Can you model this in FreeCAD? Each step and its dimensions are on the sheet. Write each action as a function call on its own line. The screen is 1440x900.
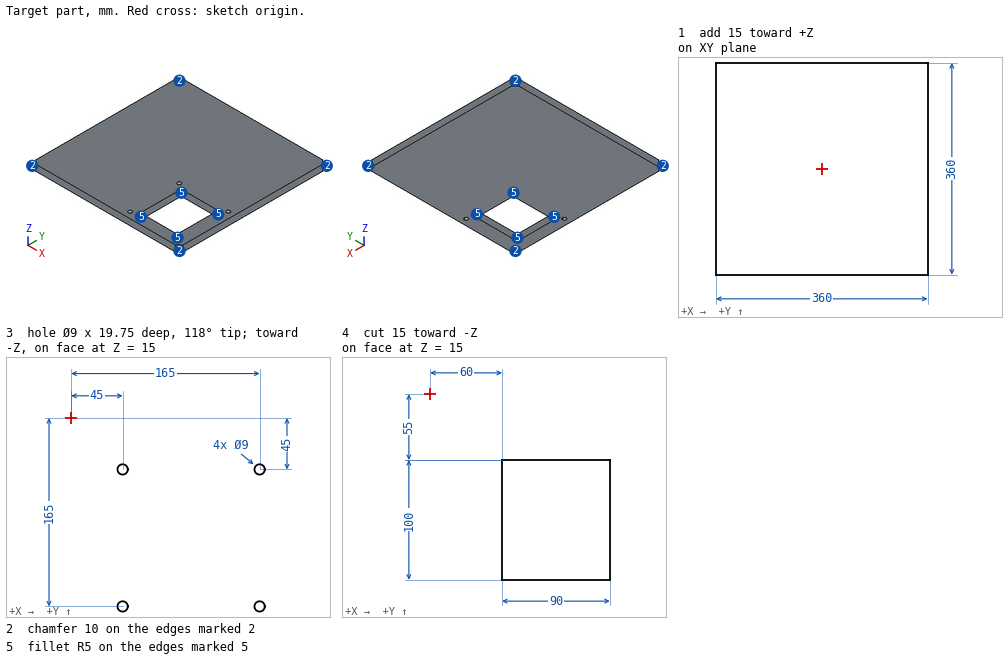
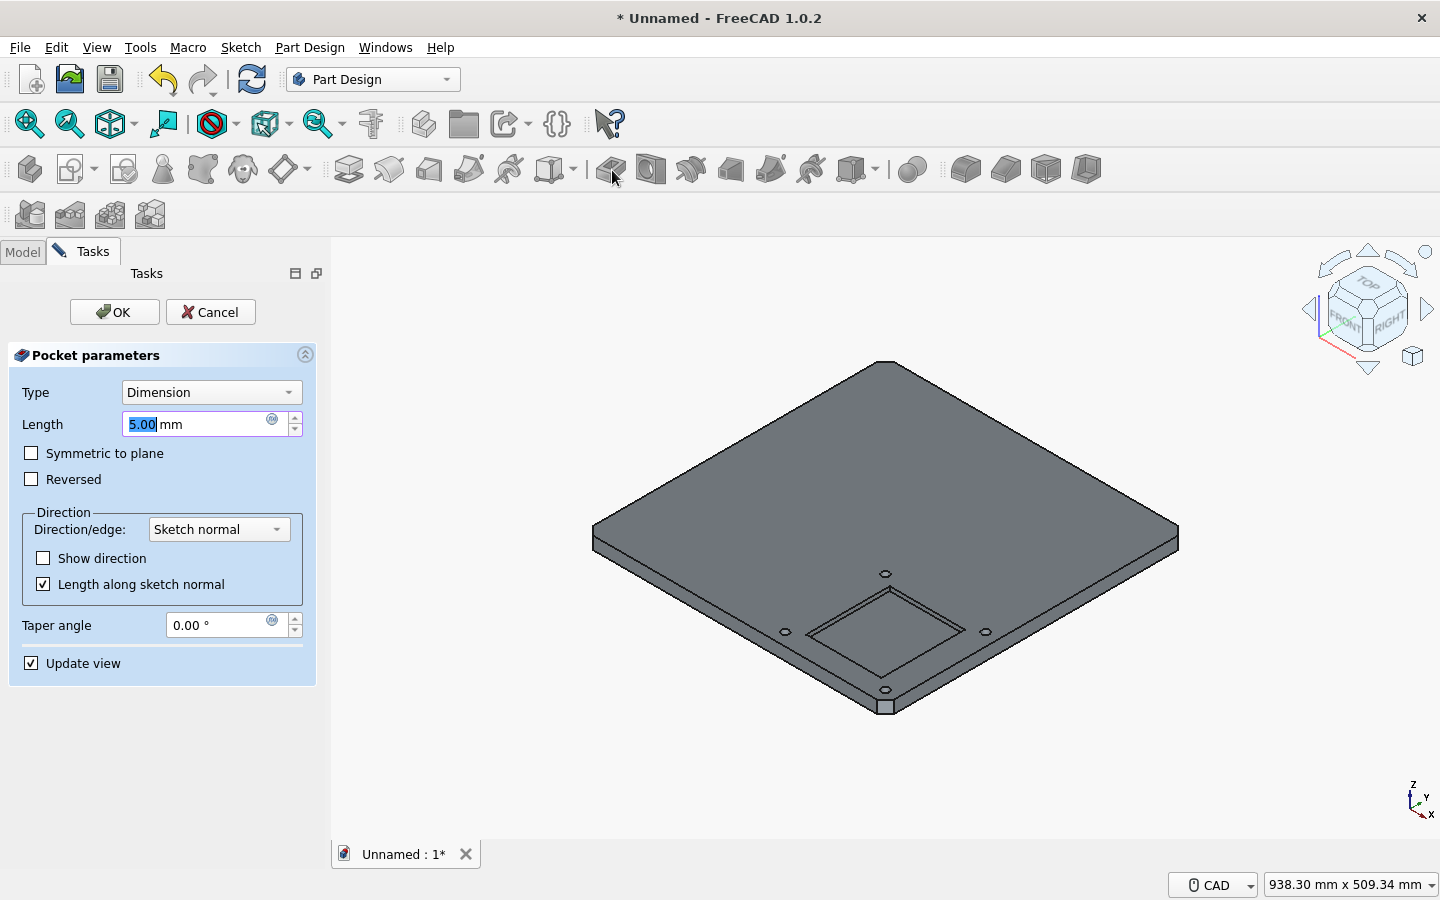
text(15)
key(Tab)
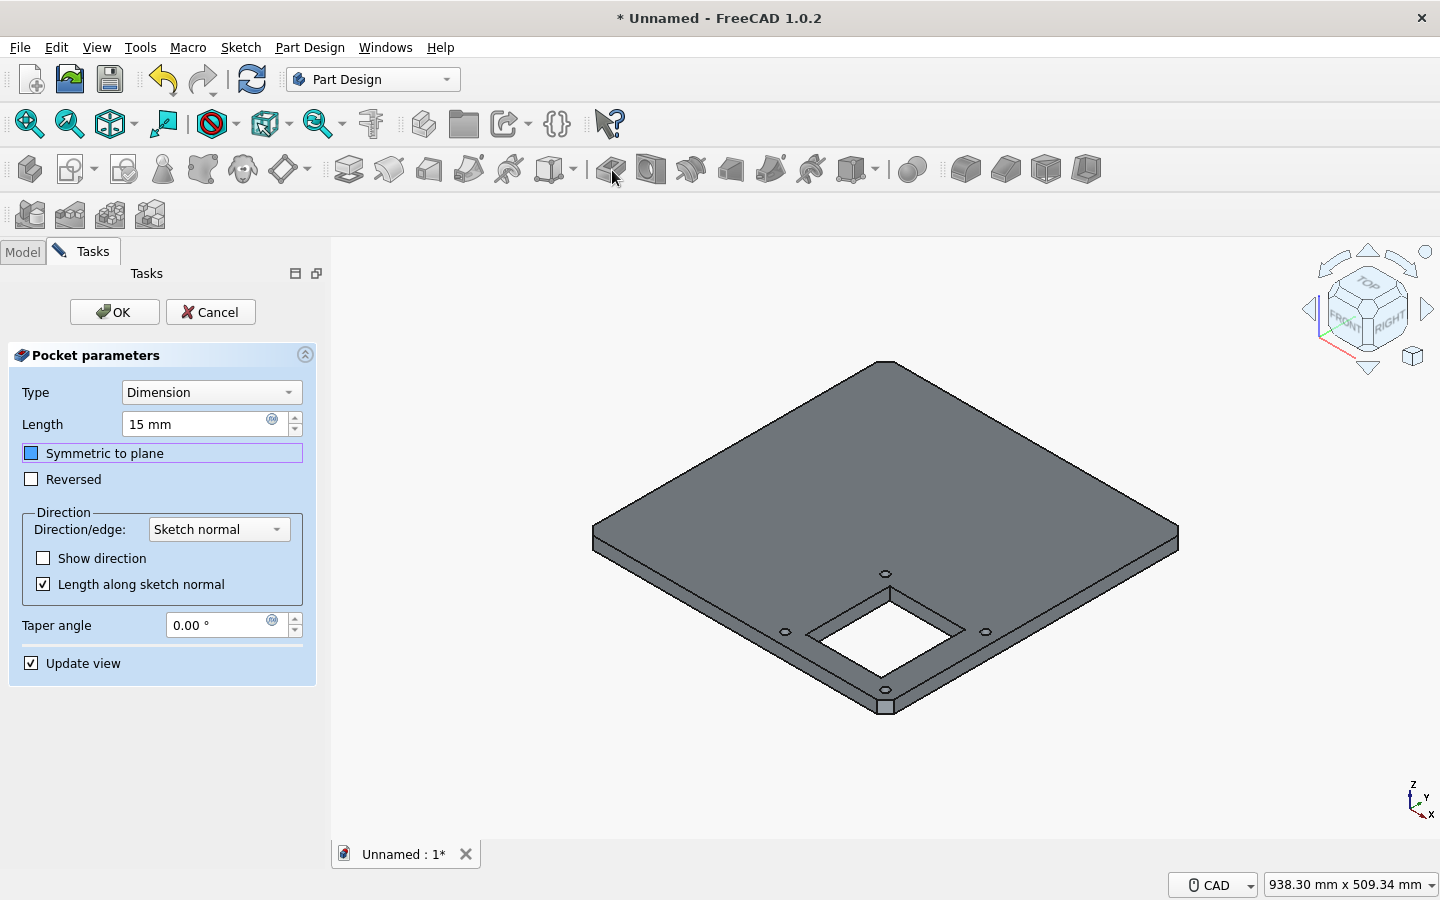
click(115, 312)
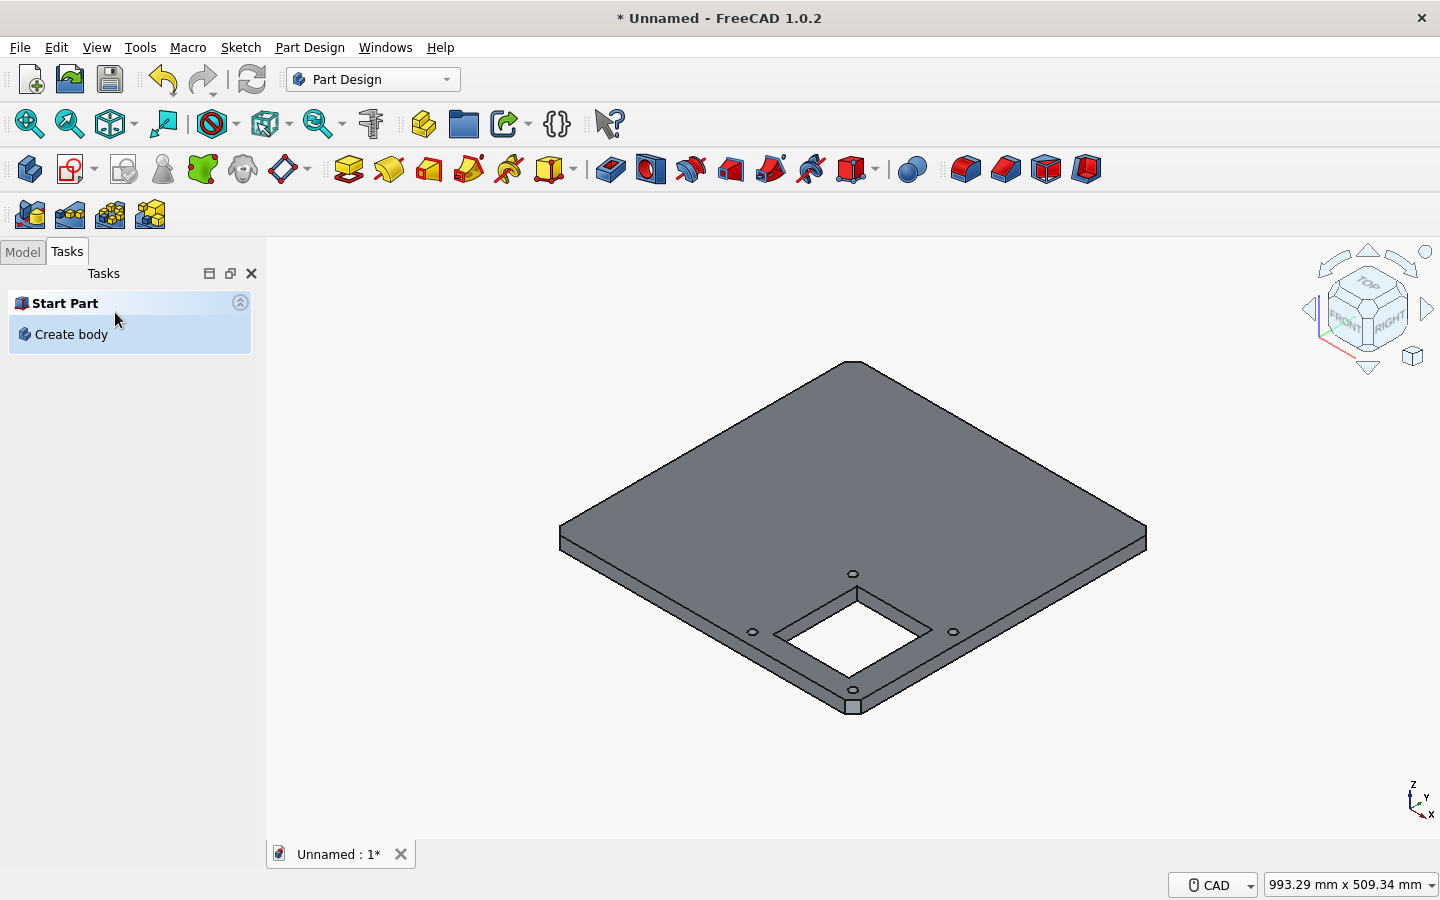
scroll(932, 636, up, 5)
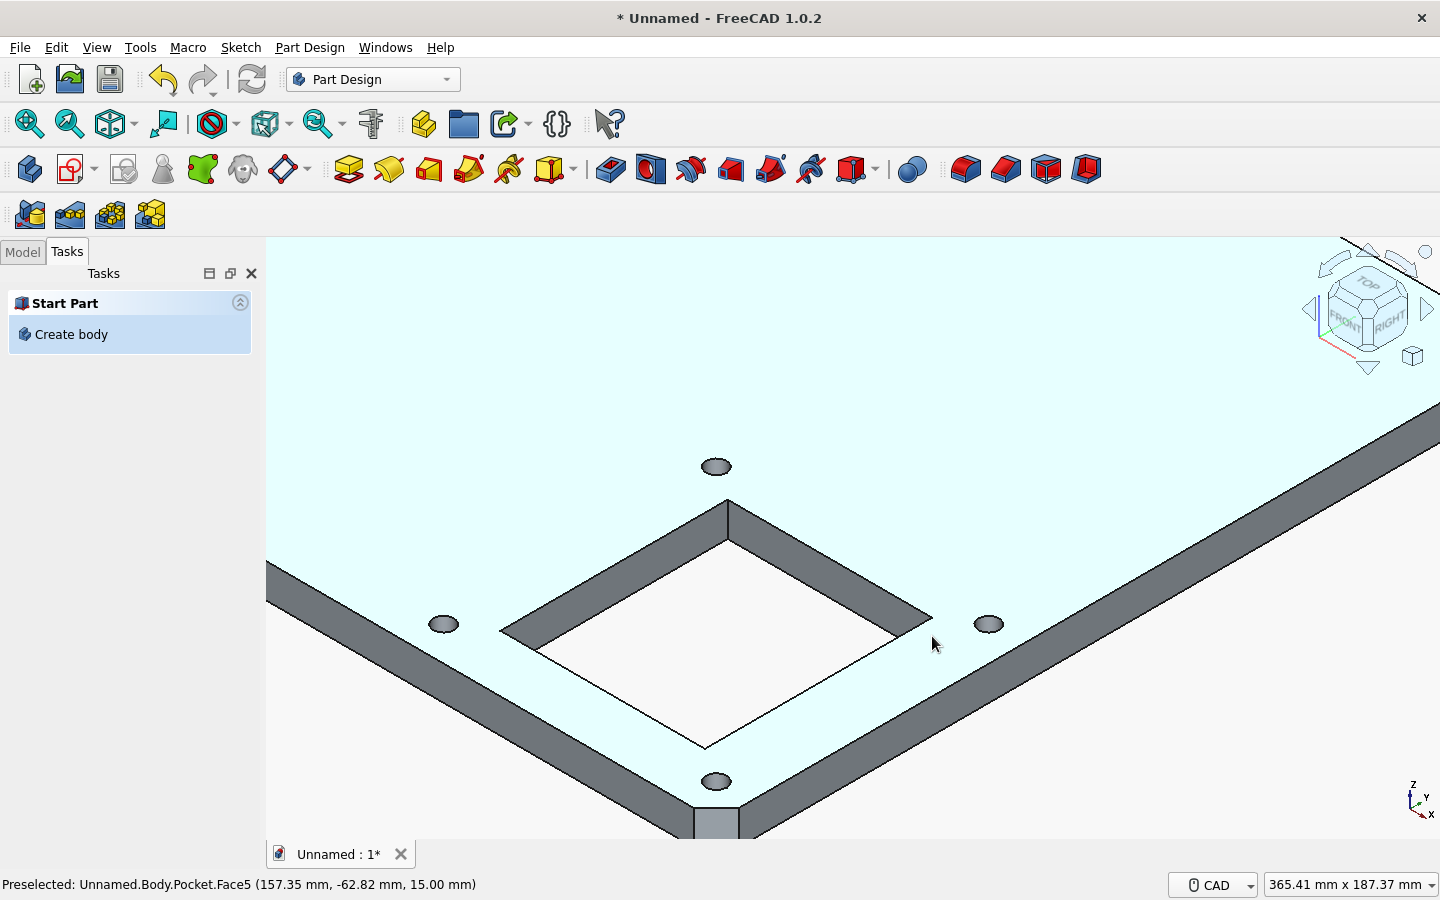
key(v)
key(f)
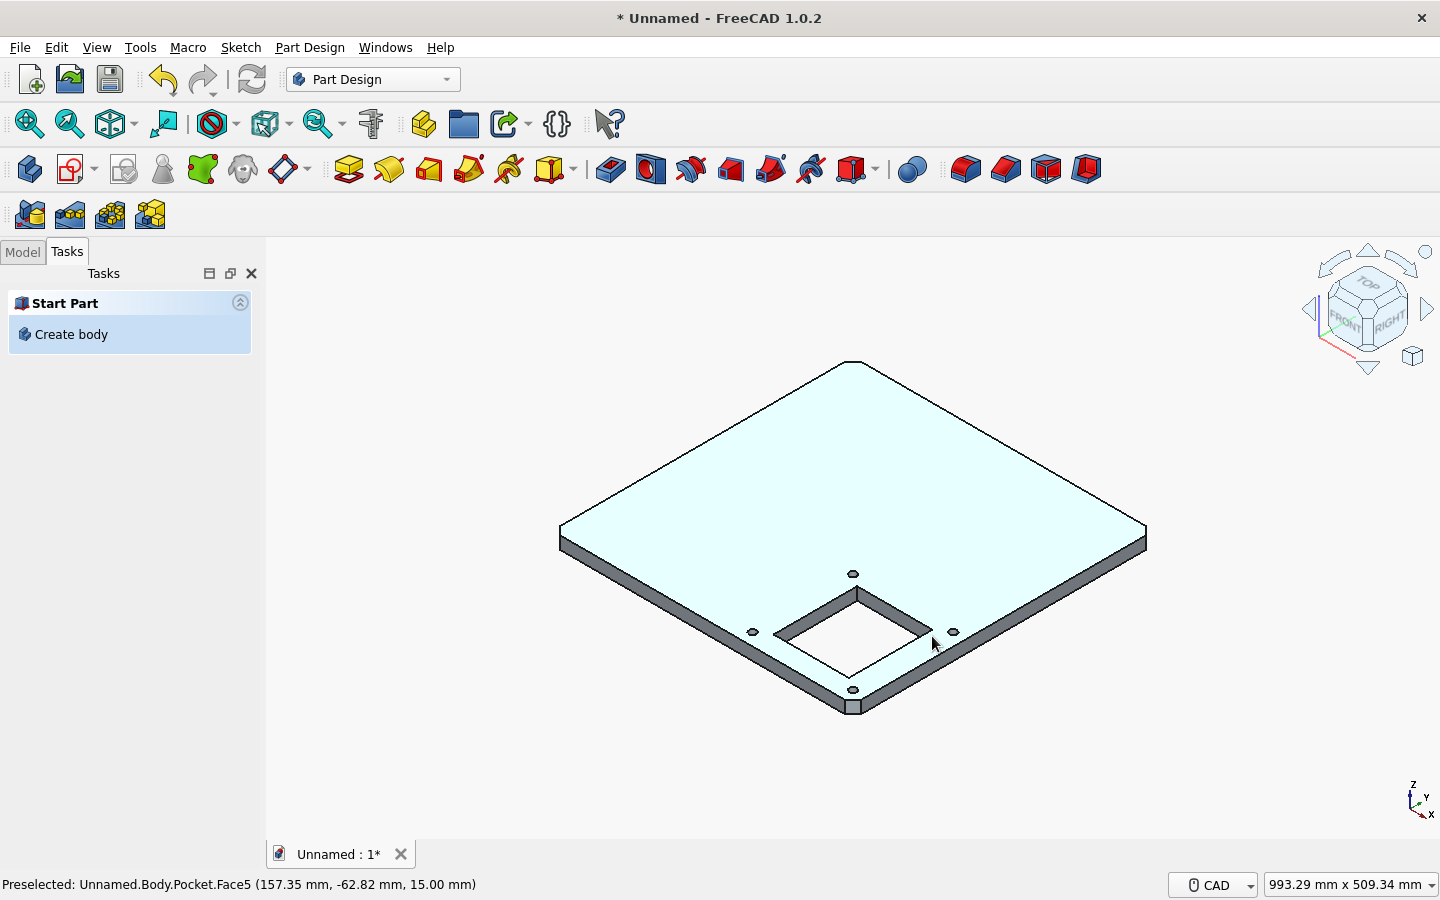
key(2)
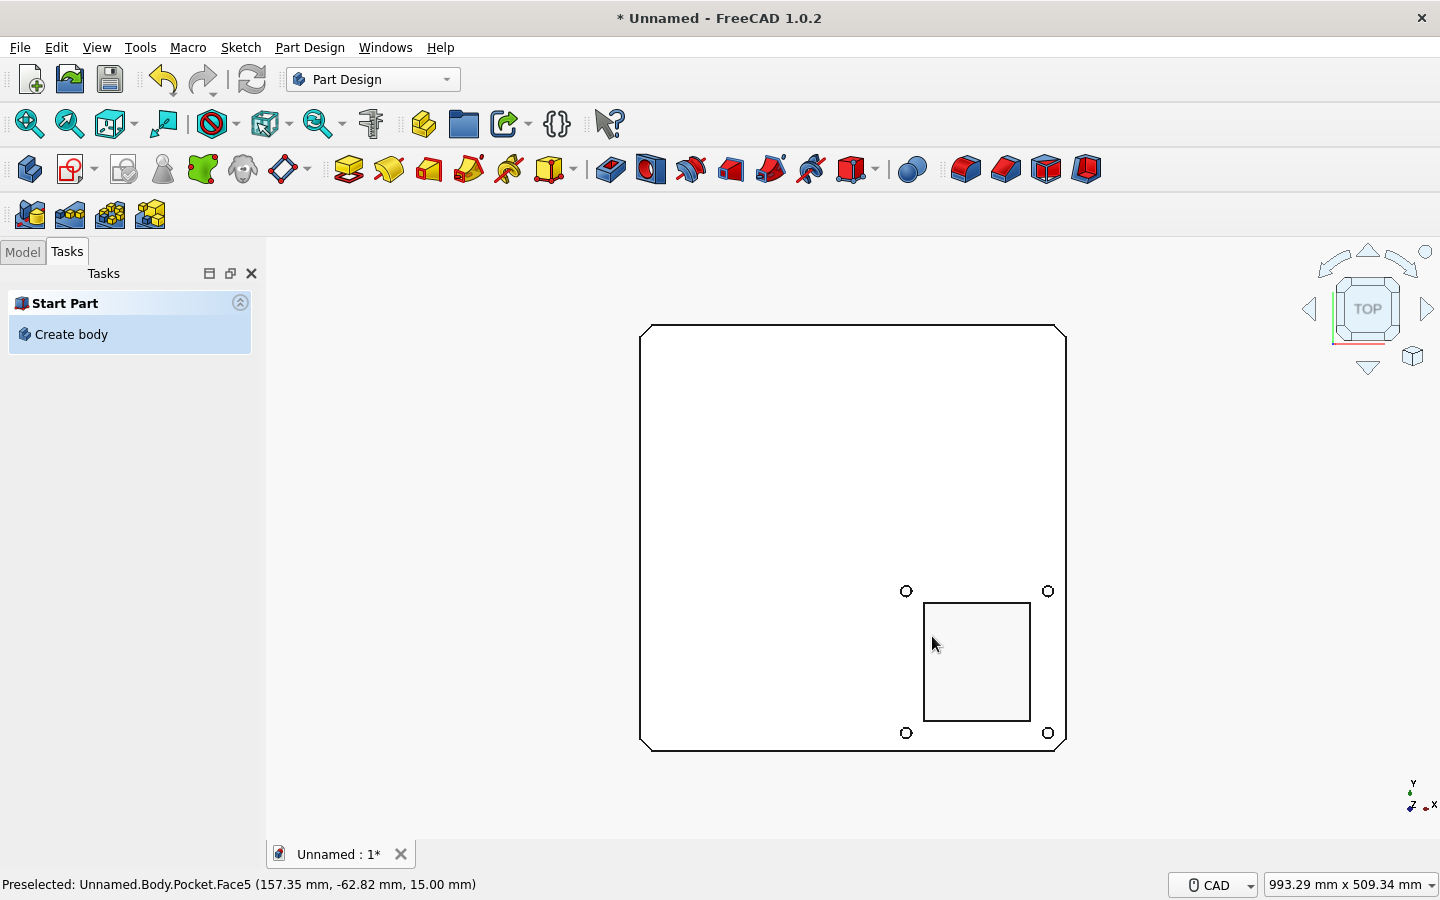
scroll(1030, 602, up, 5)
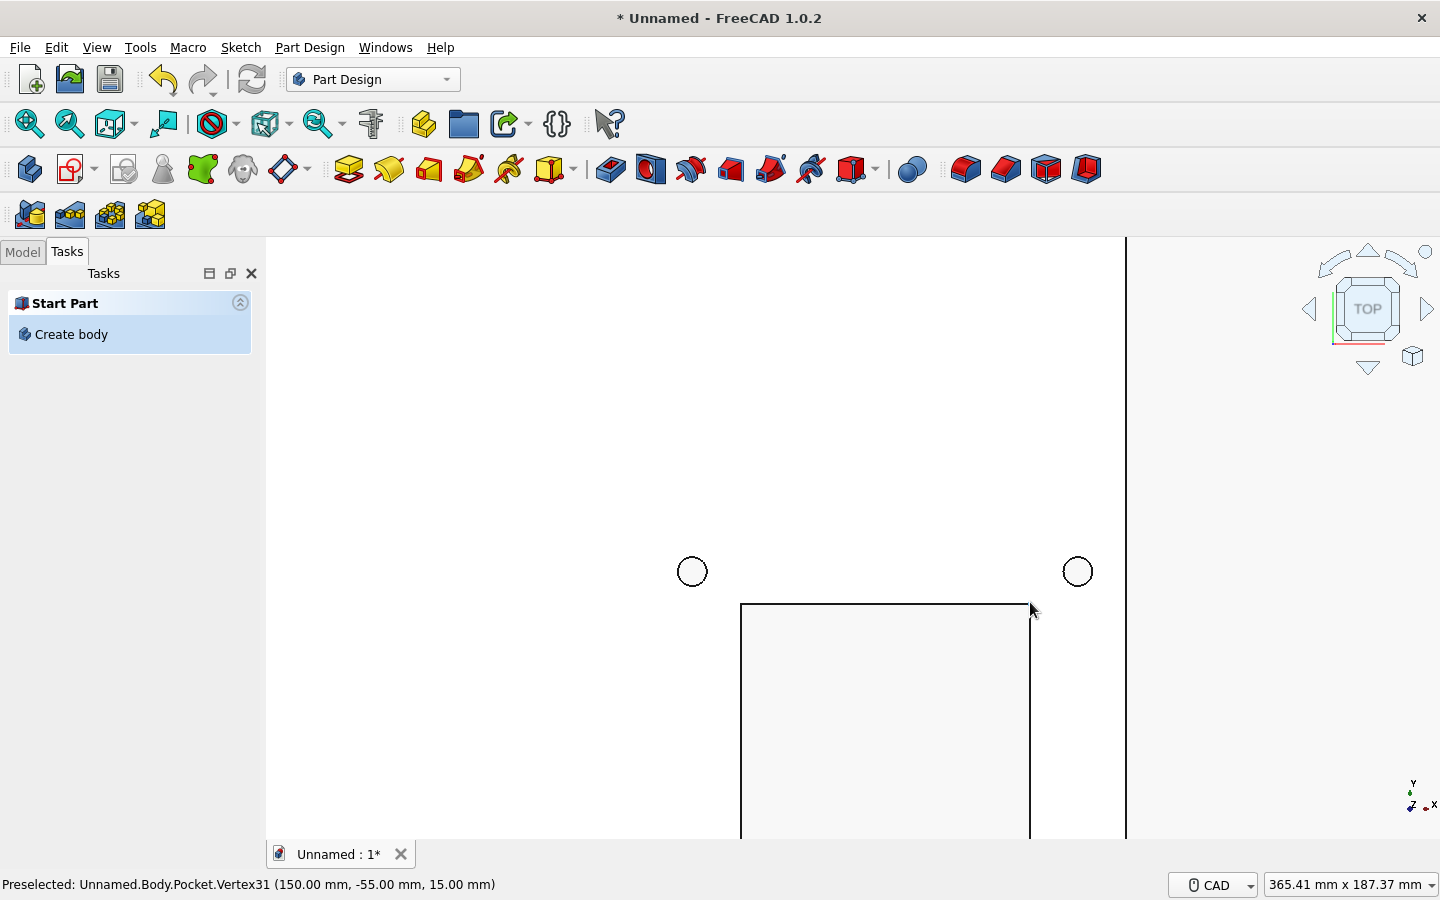
key(v)
key(f)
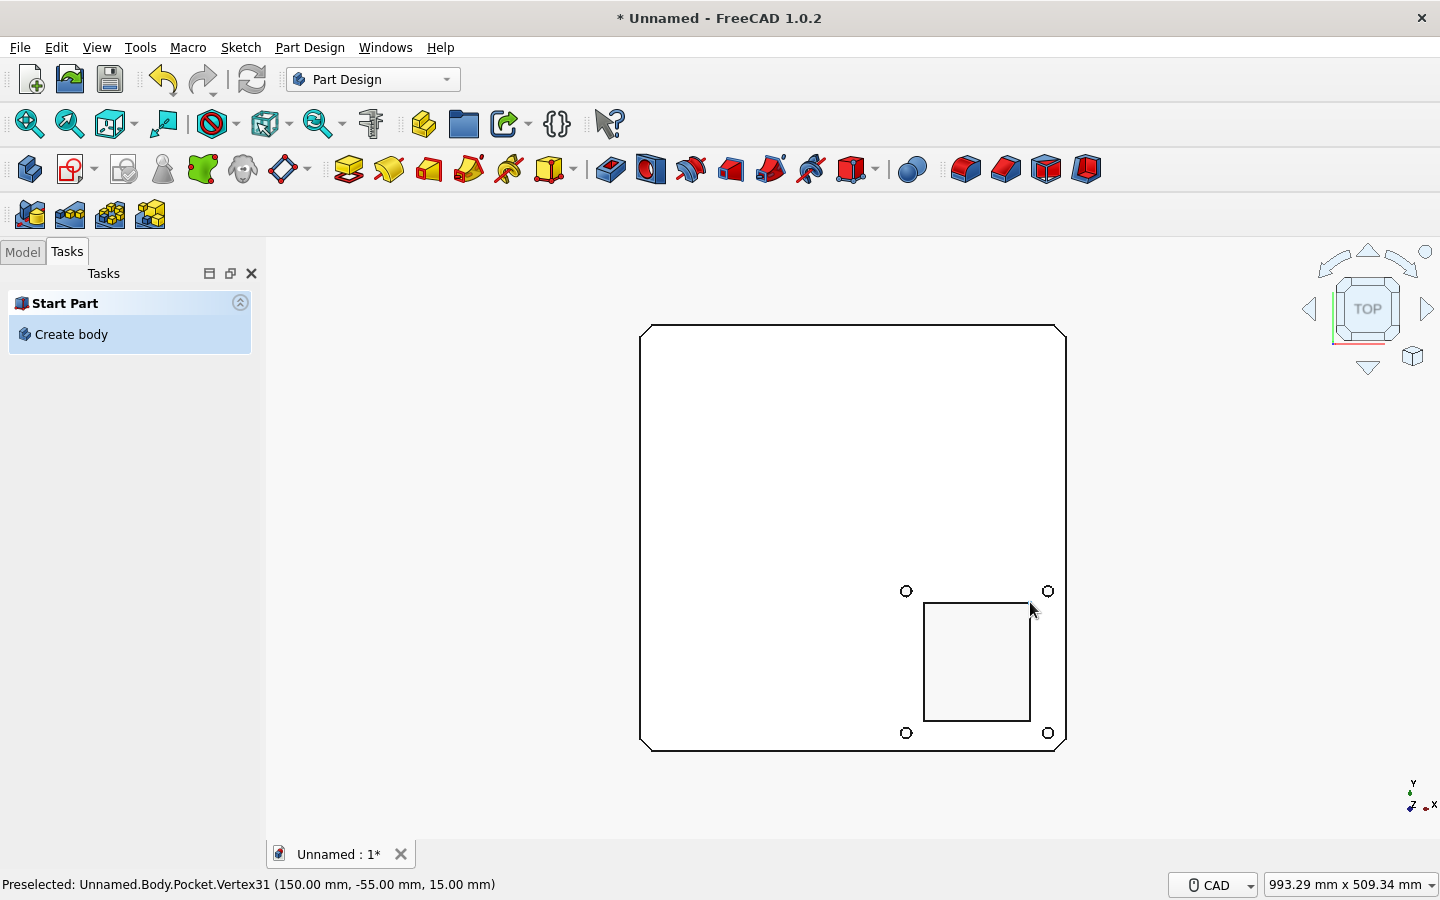
key(0)